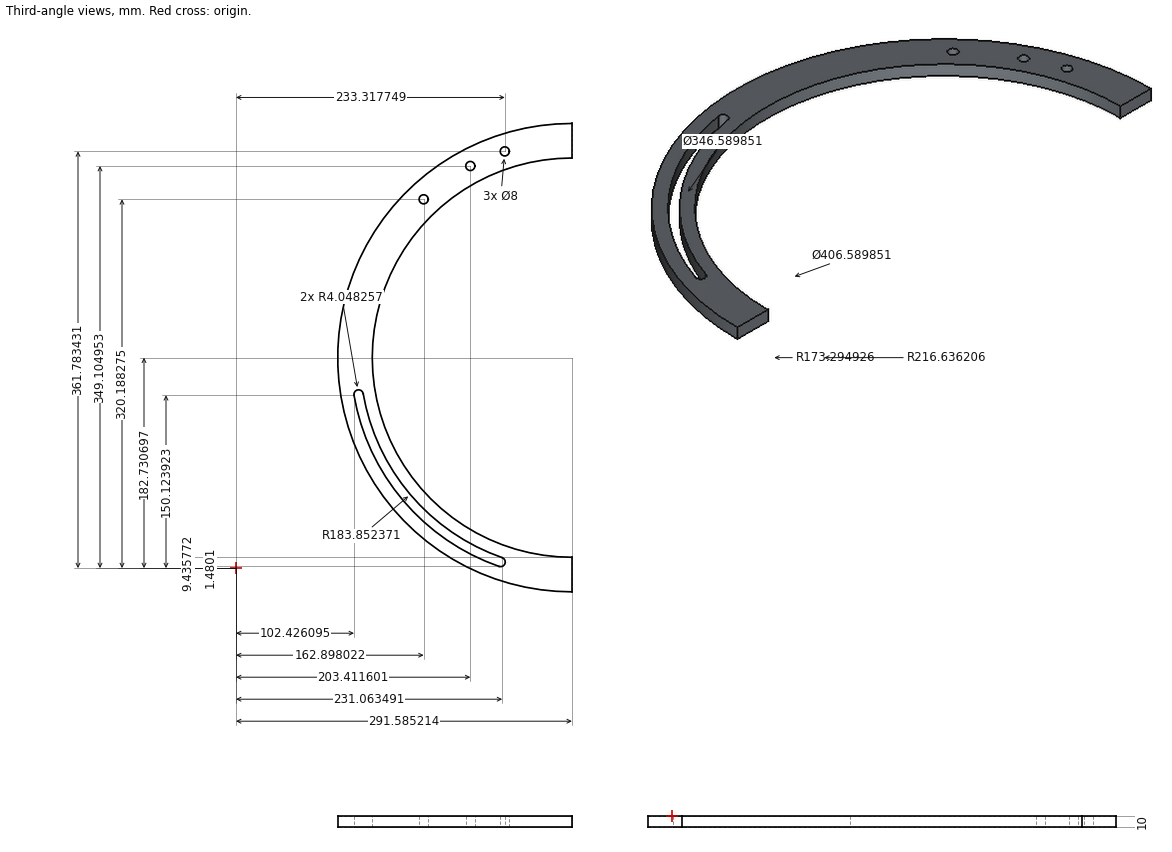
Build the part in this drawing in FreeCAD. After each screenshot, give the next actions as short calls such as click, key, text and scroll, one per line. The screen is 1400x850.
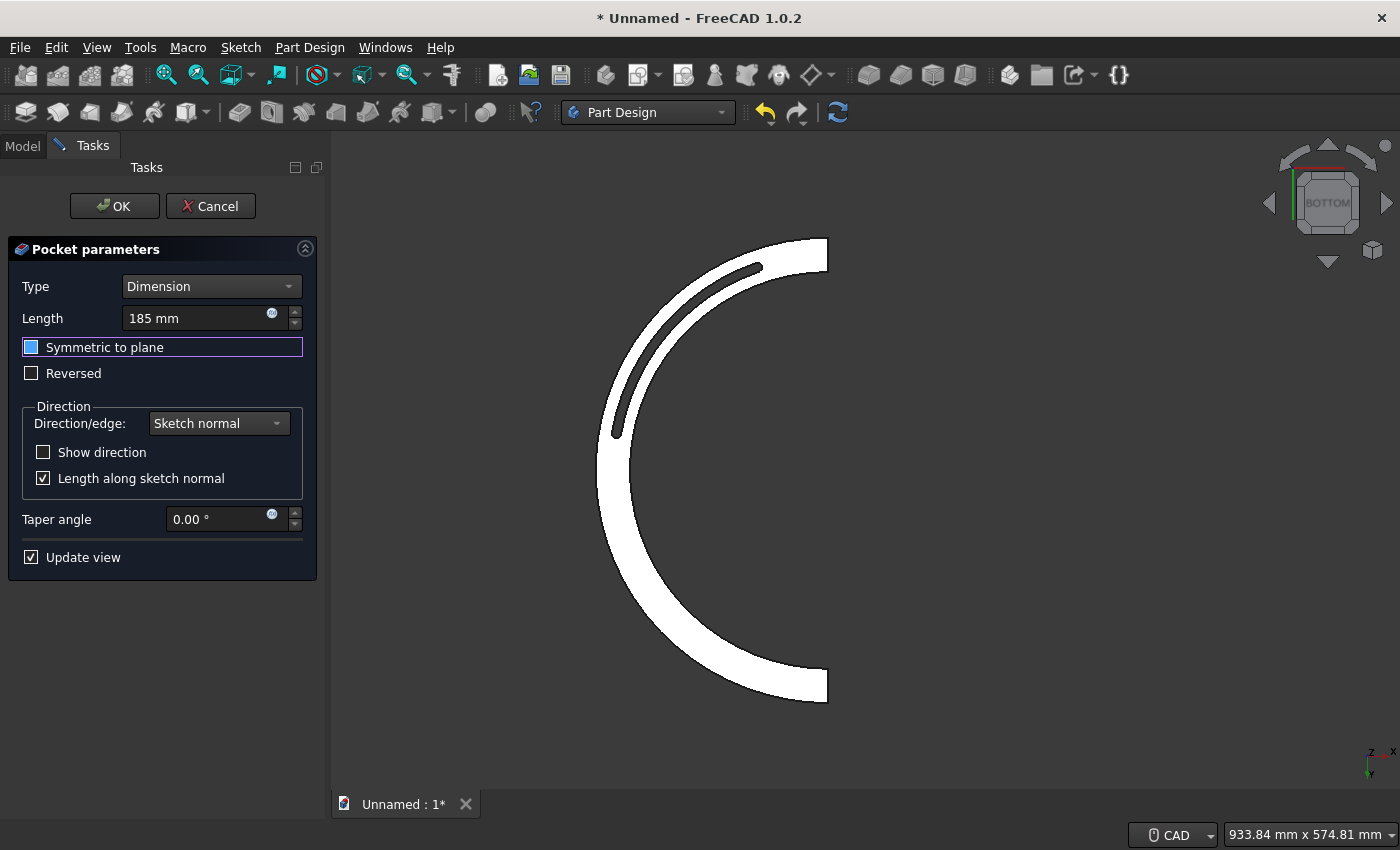
click(115, 206)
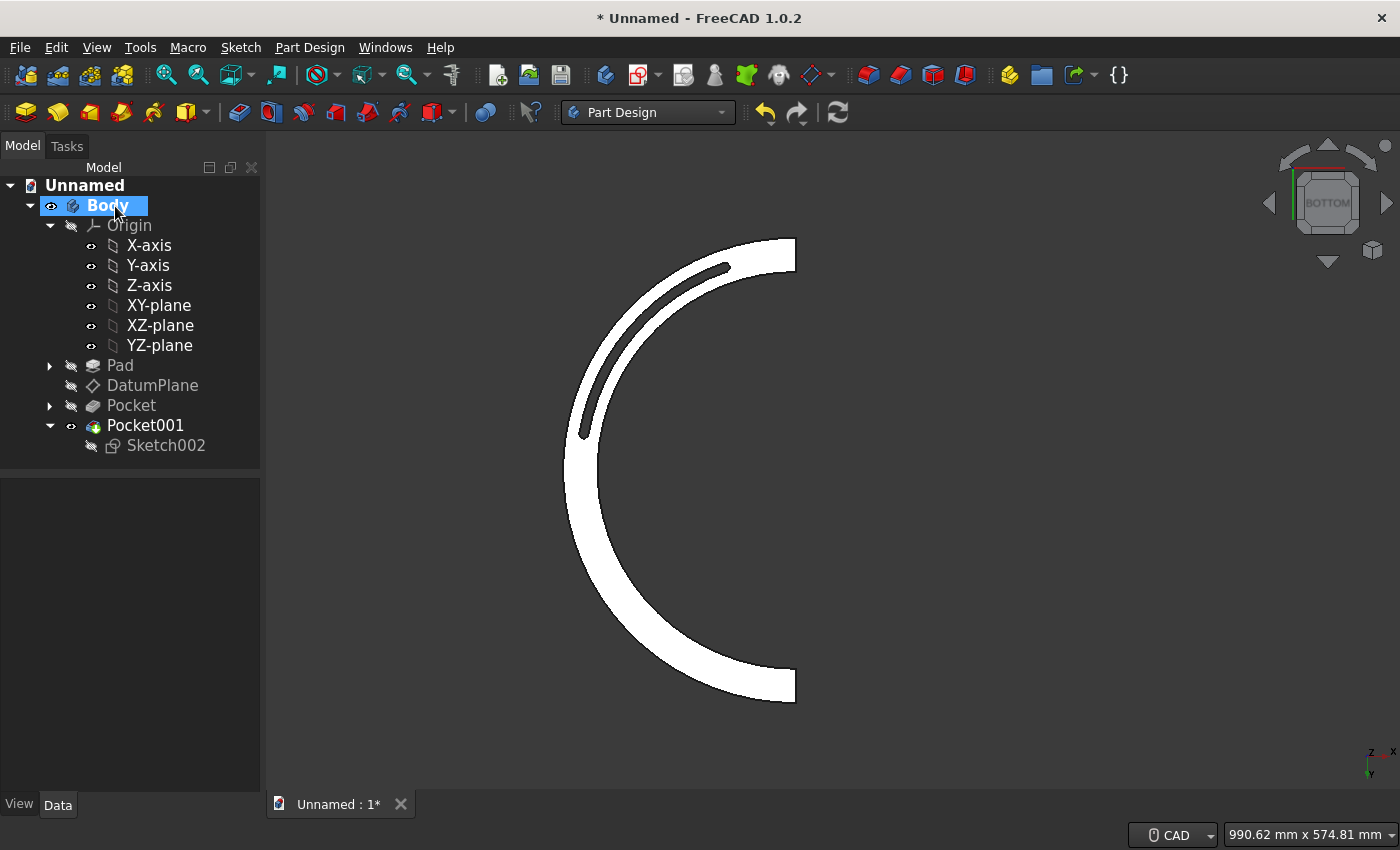
key(0)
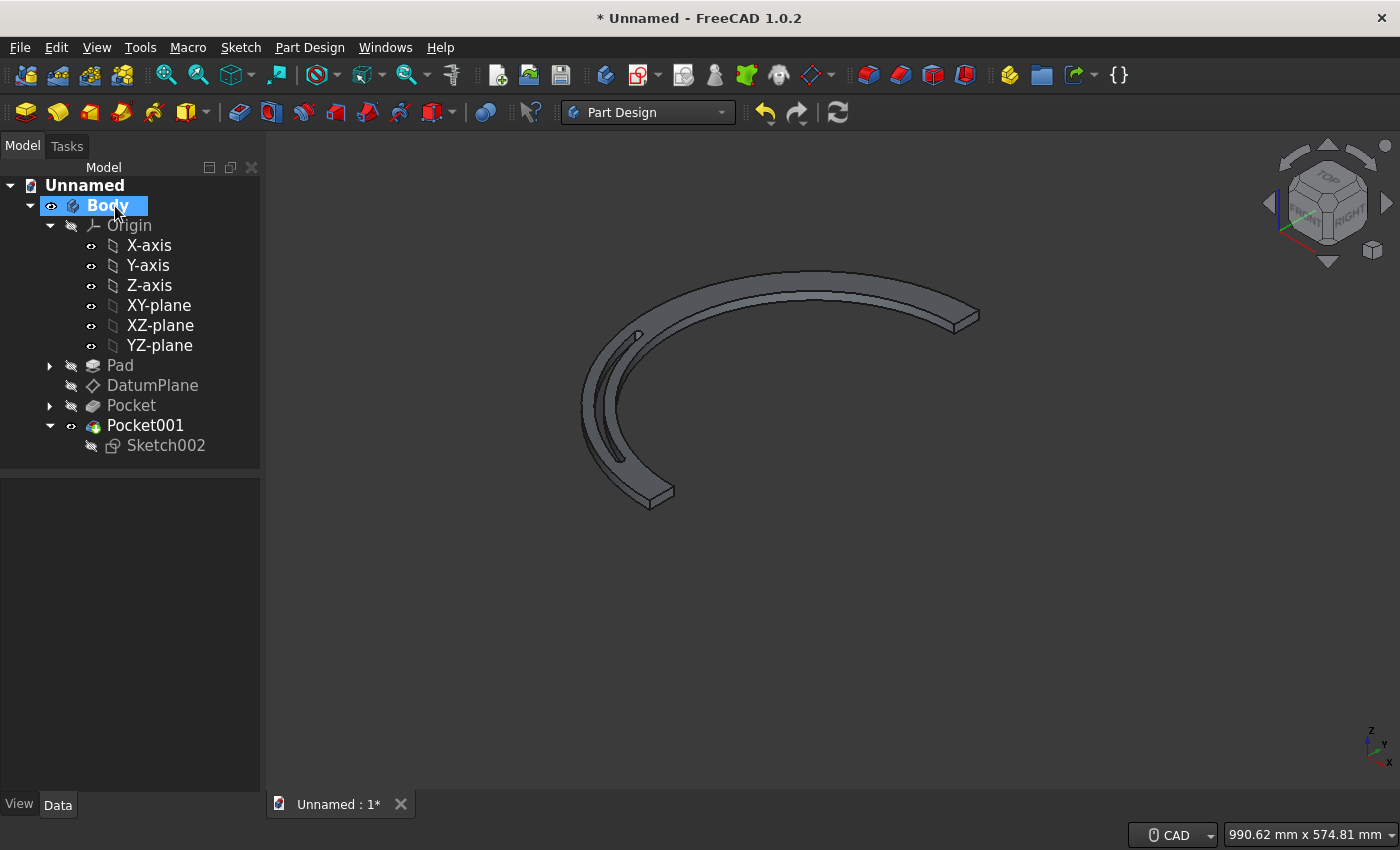
key(v)
key(f)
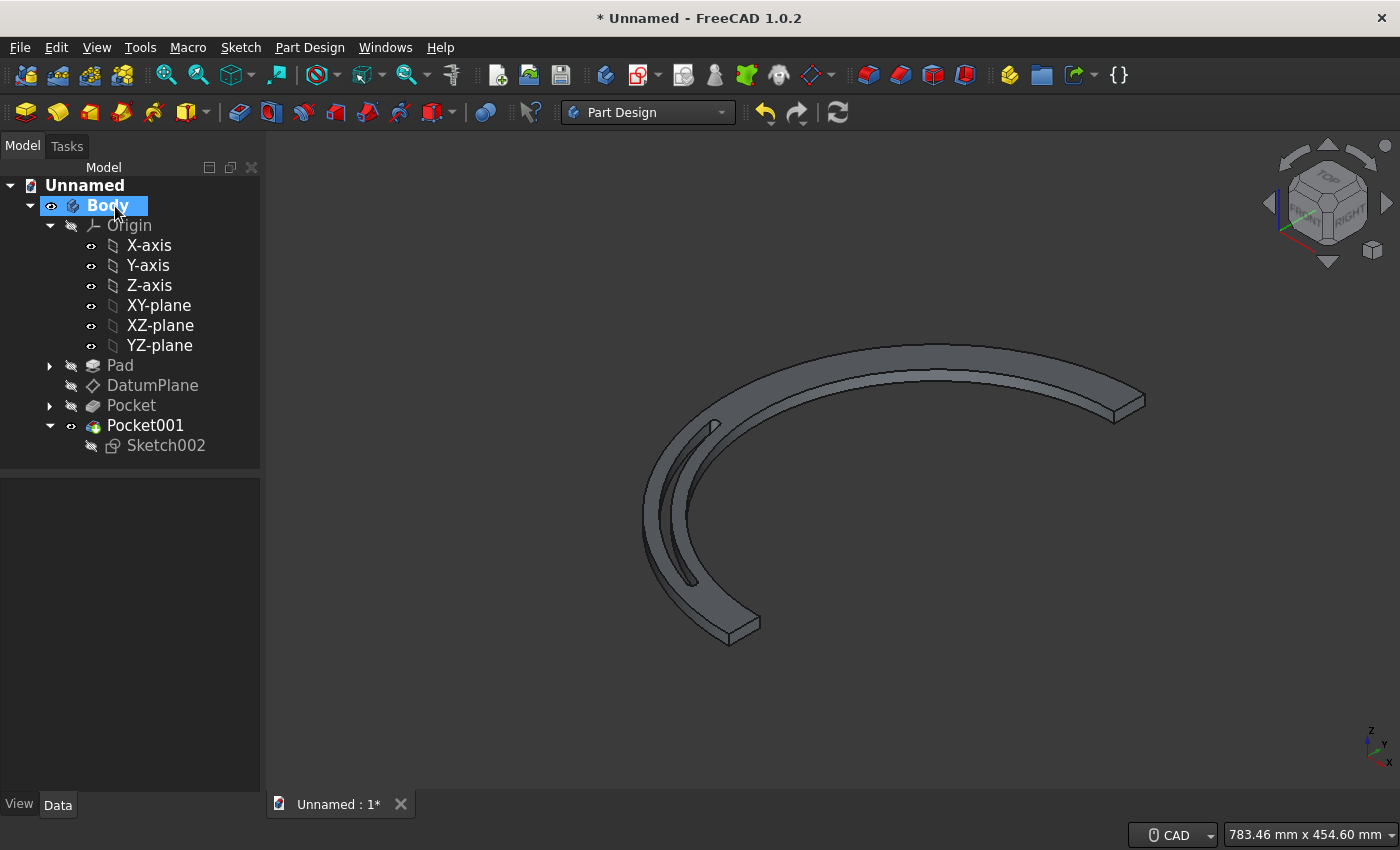
click(1041, 367)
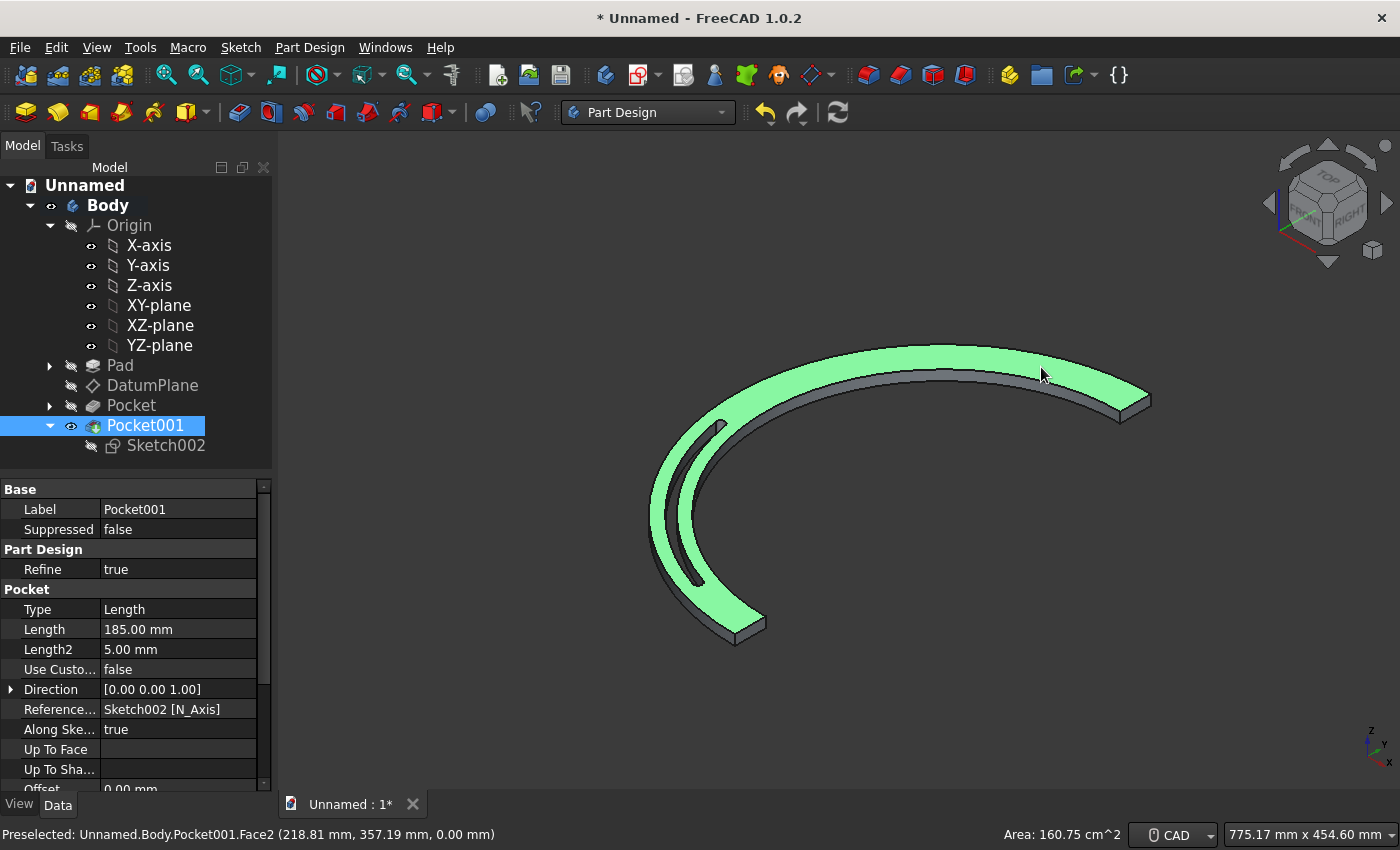
click(638, 76)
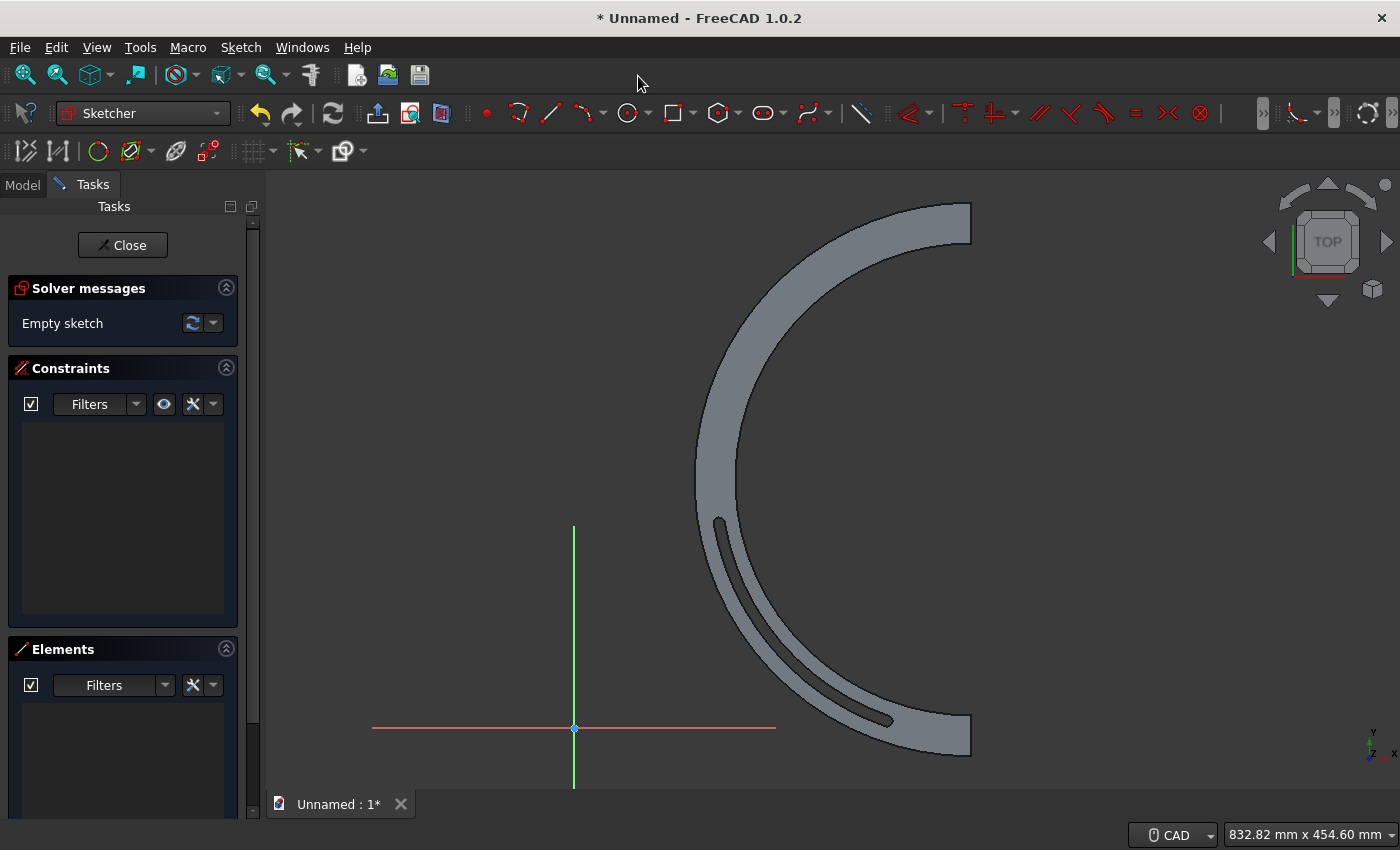
scroll(860, 221, up, 9)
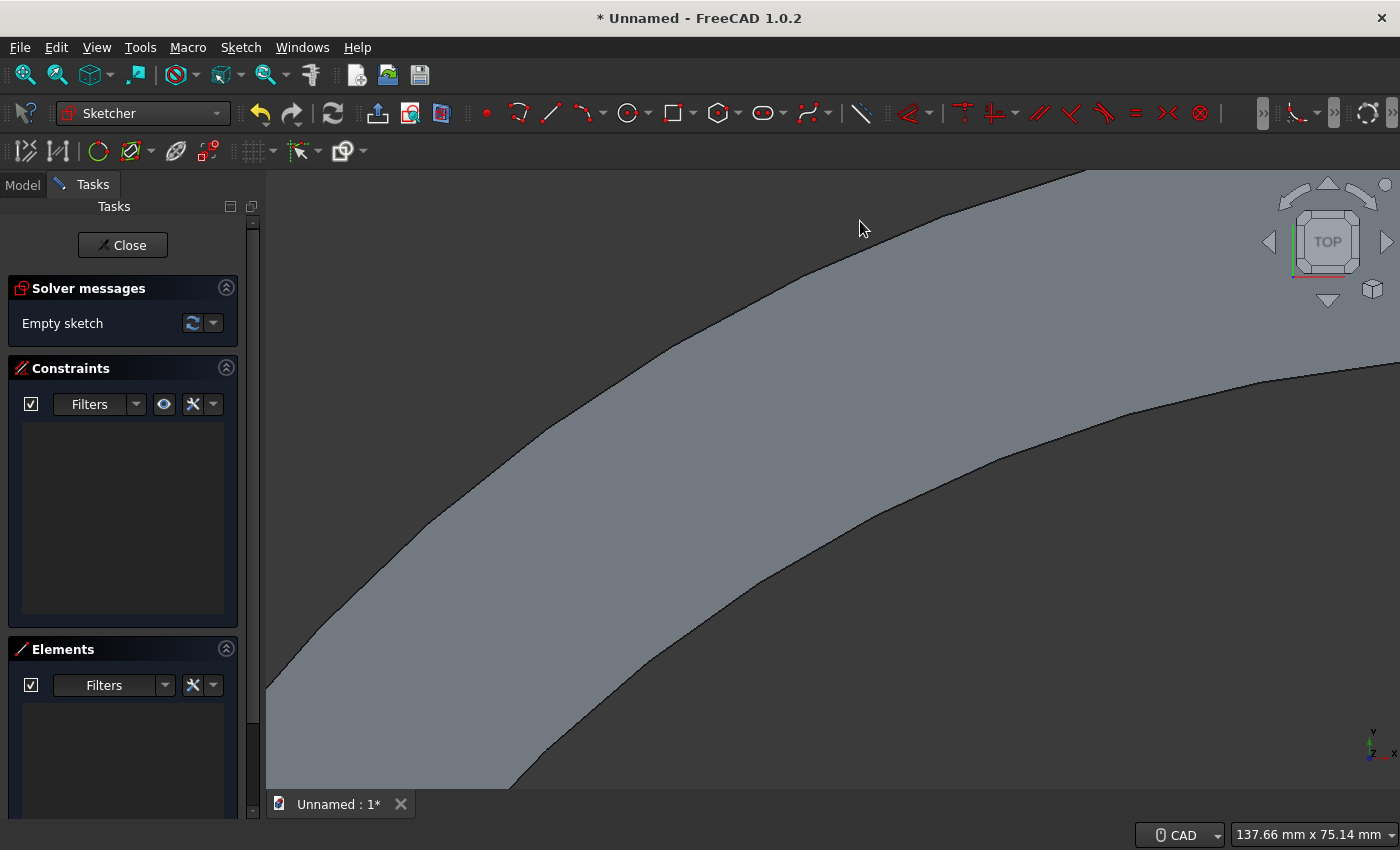
click(628, 114)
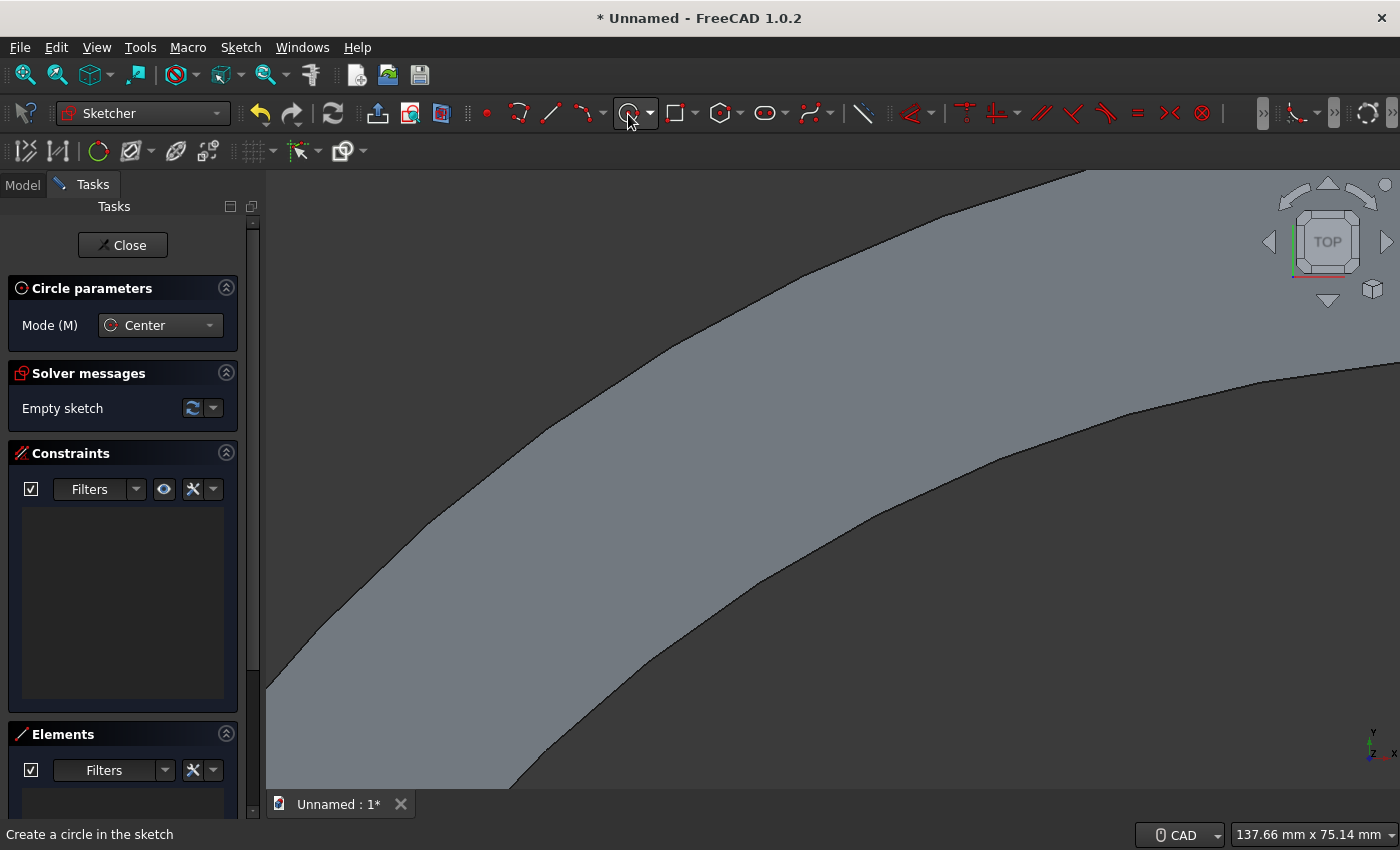
click(1051, 309)
move(1074, 286)